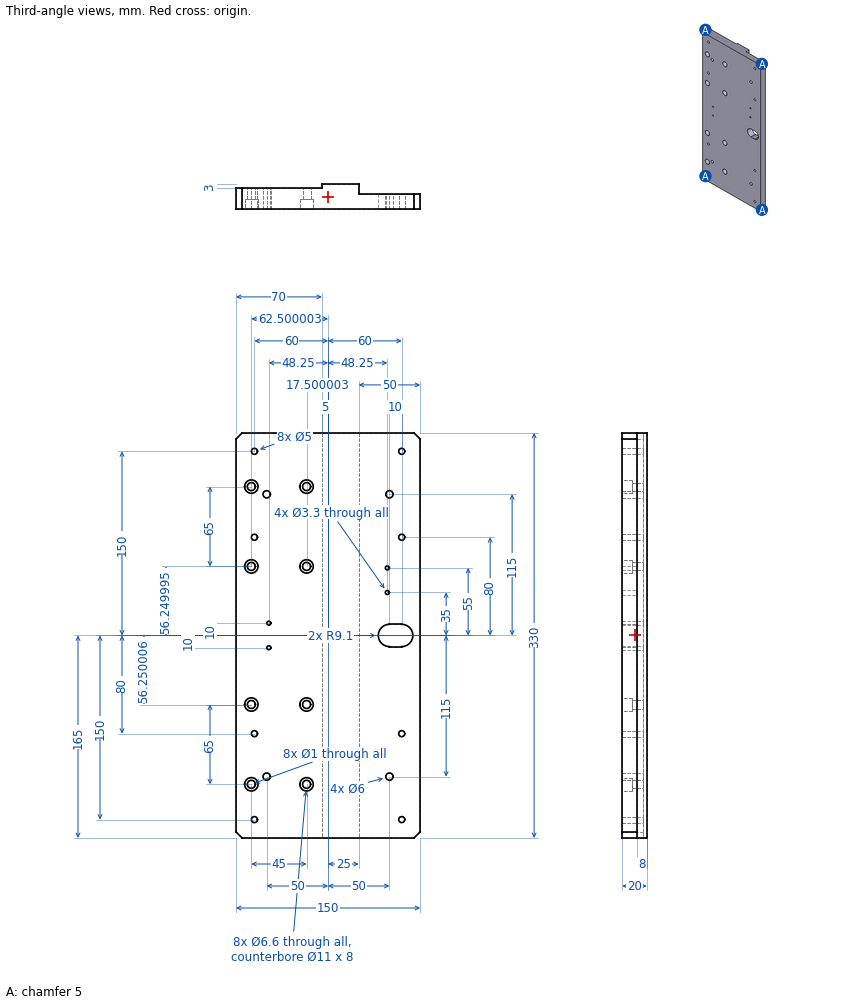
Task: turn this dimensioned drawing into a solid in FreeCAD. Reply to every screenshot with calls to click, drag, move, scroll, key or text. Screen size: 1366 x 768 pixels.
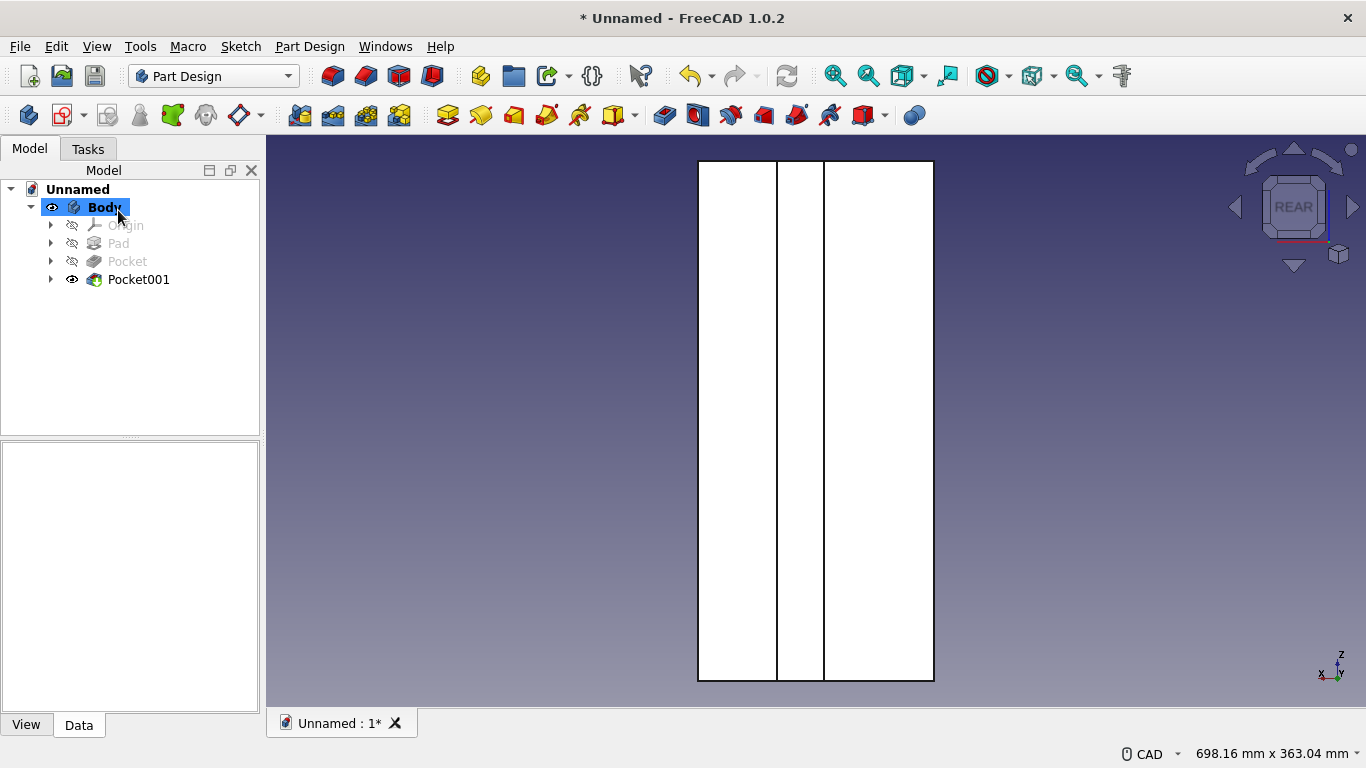
click(879, 569)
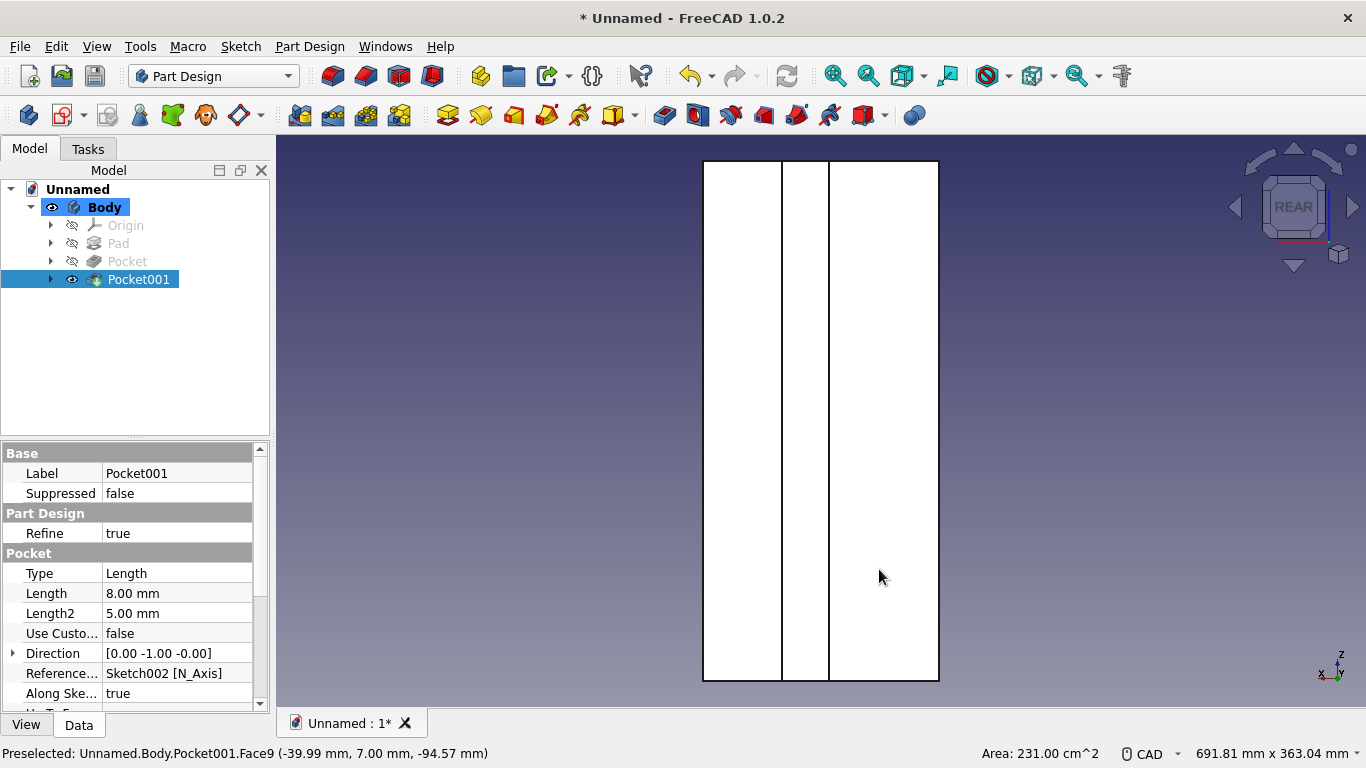
click(62, 116)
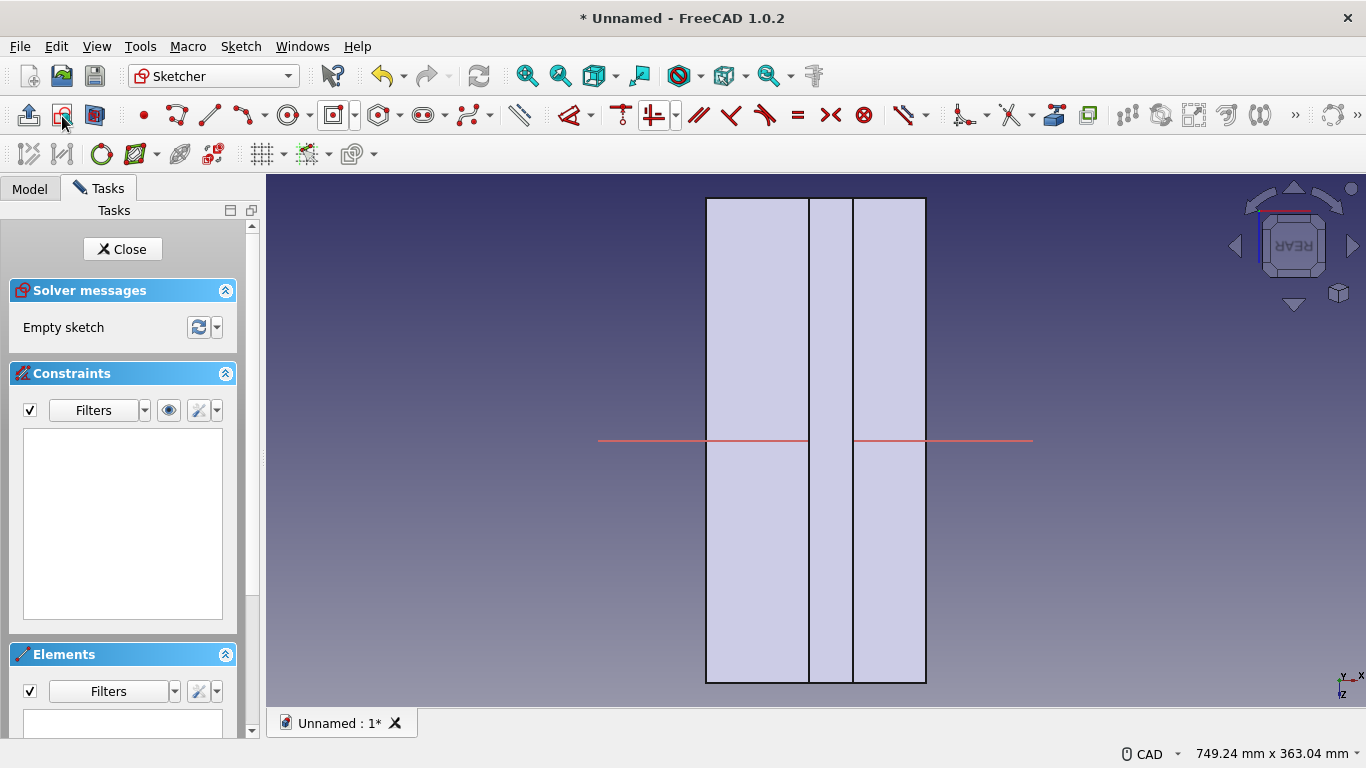
click(95, 116)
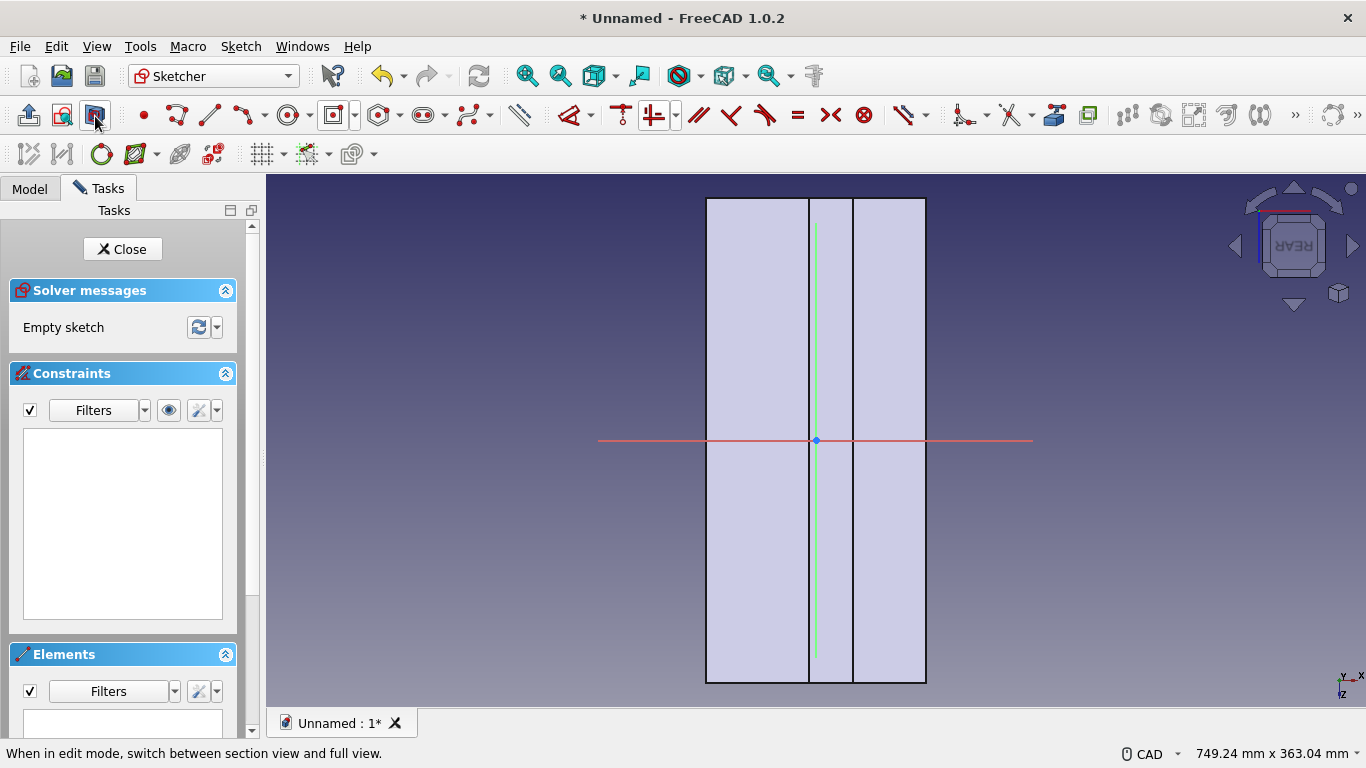
click(288, 116)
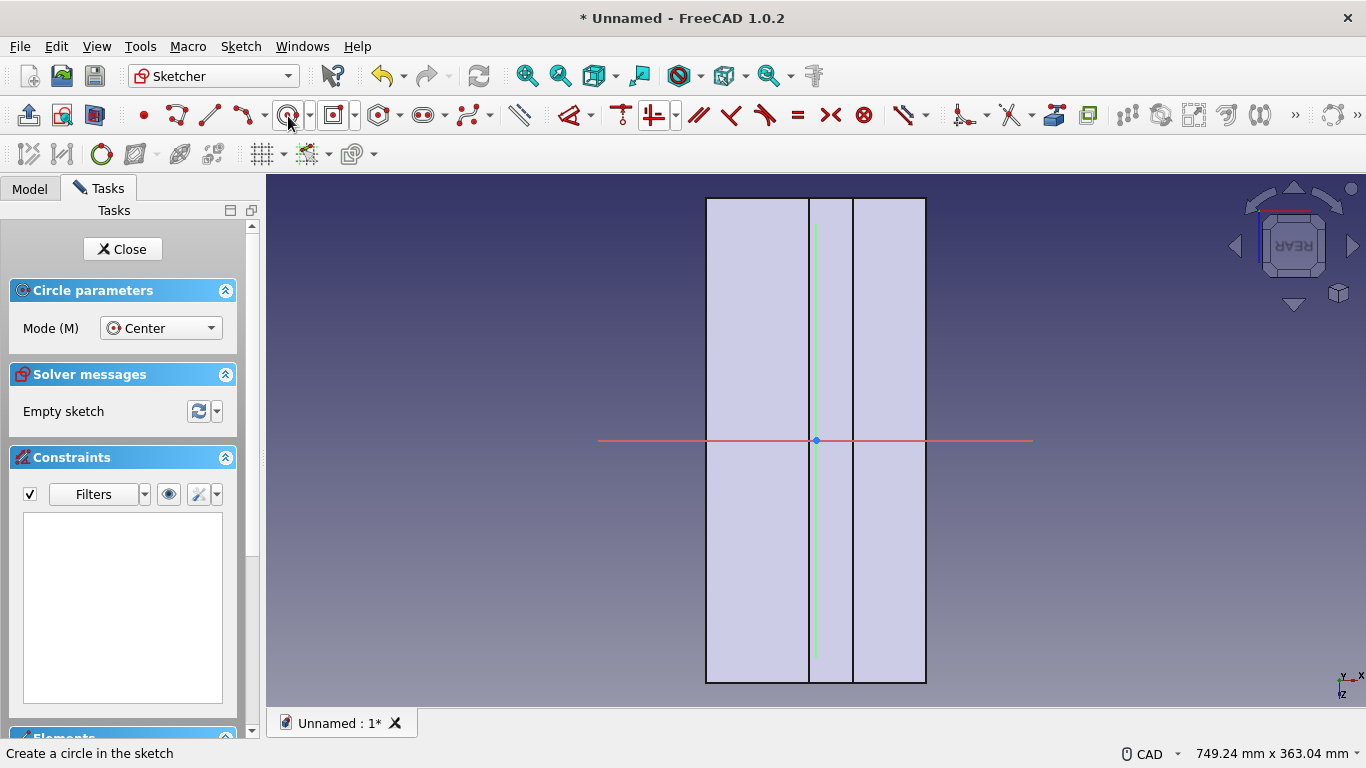
scroll(724, 262, up, 18)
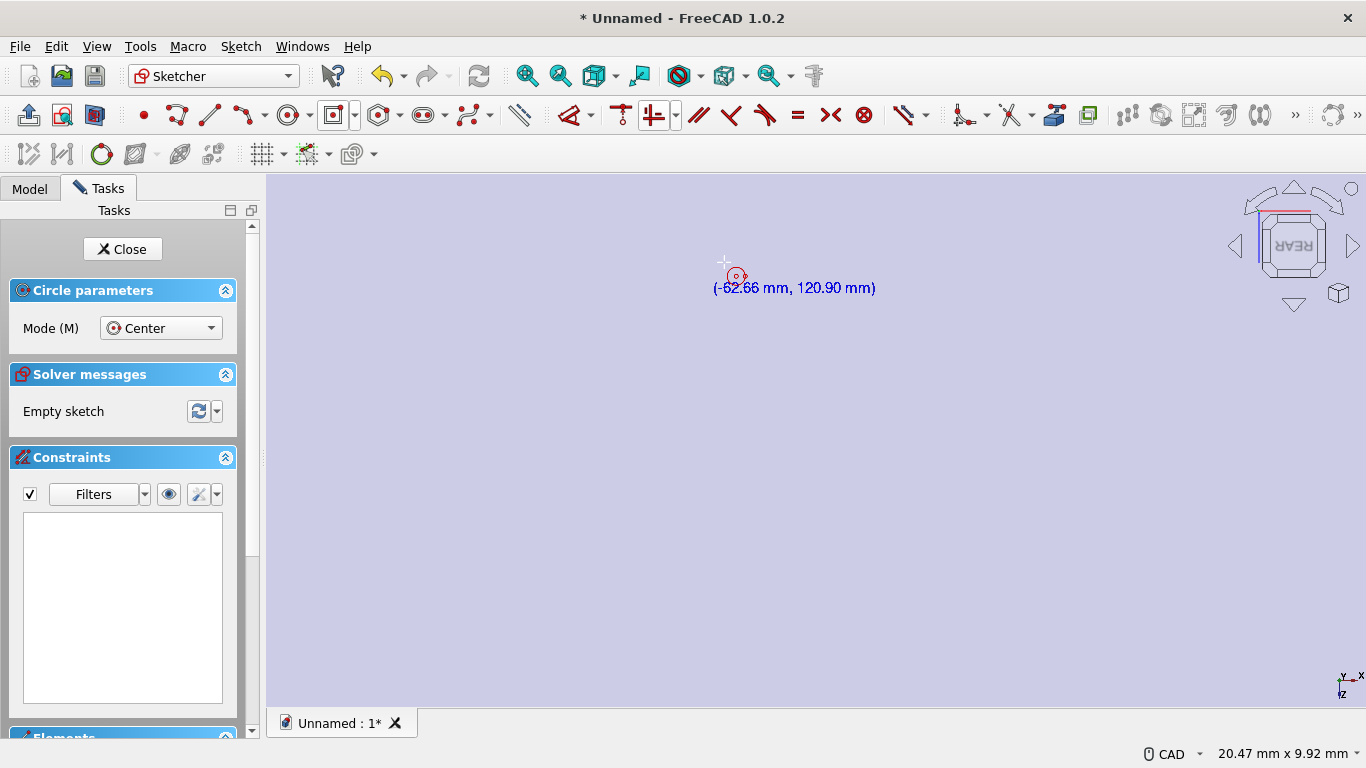
scroll(702, 262, down, 18)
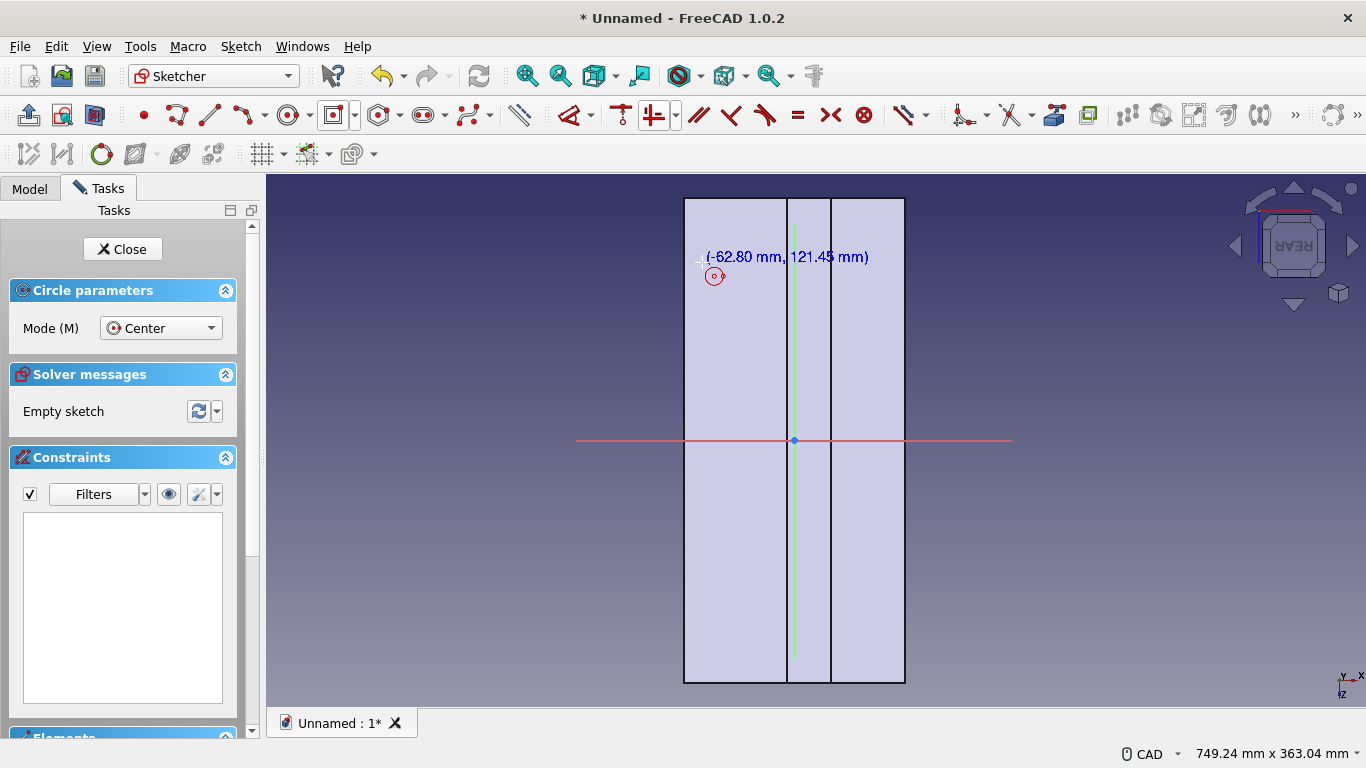
click(703, 262)
move(703, 262)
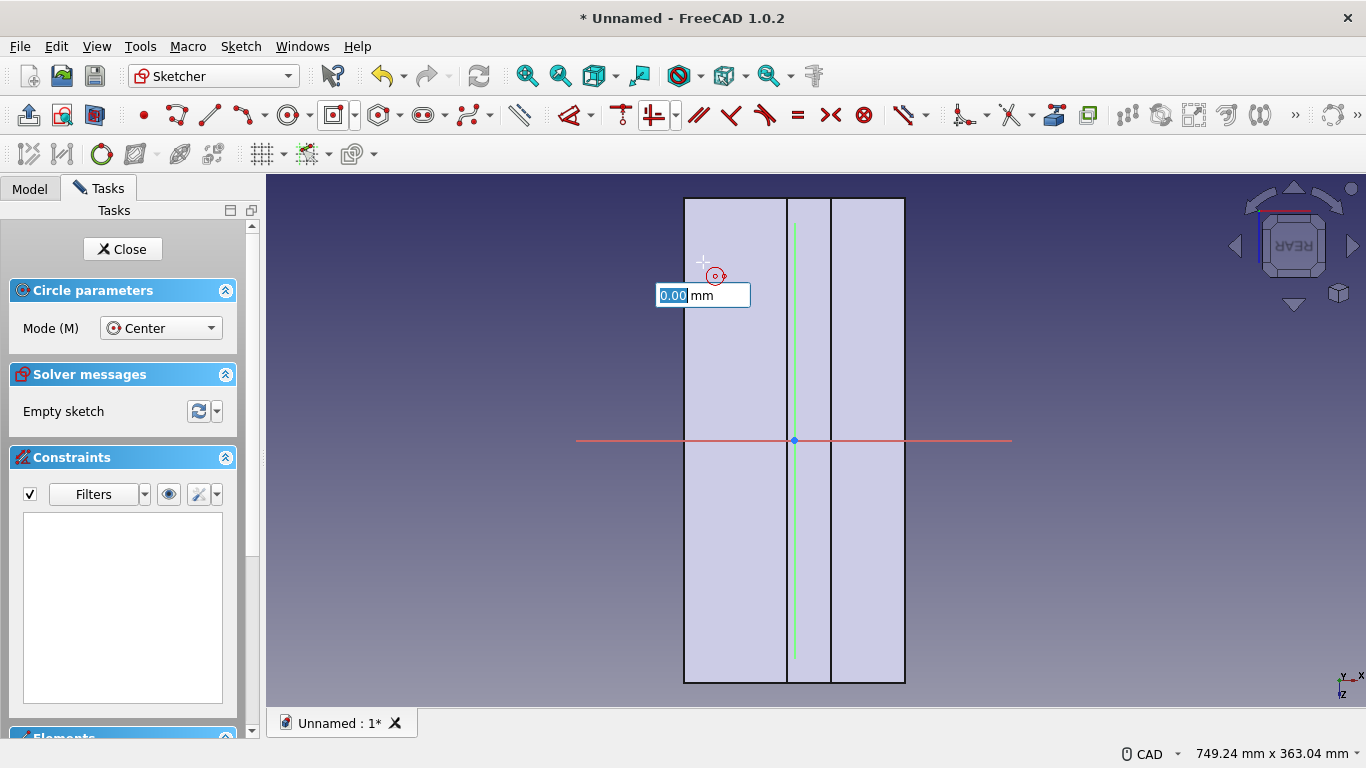
text(1)
key(Return)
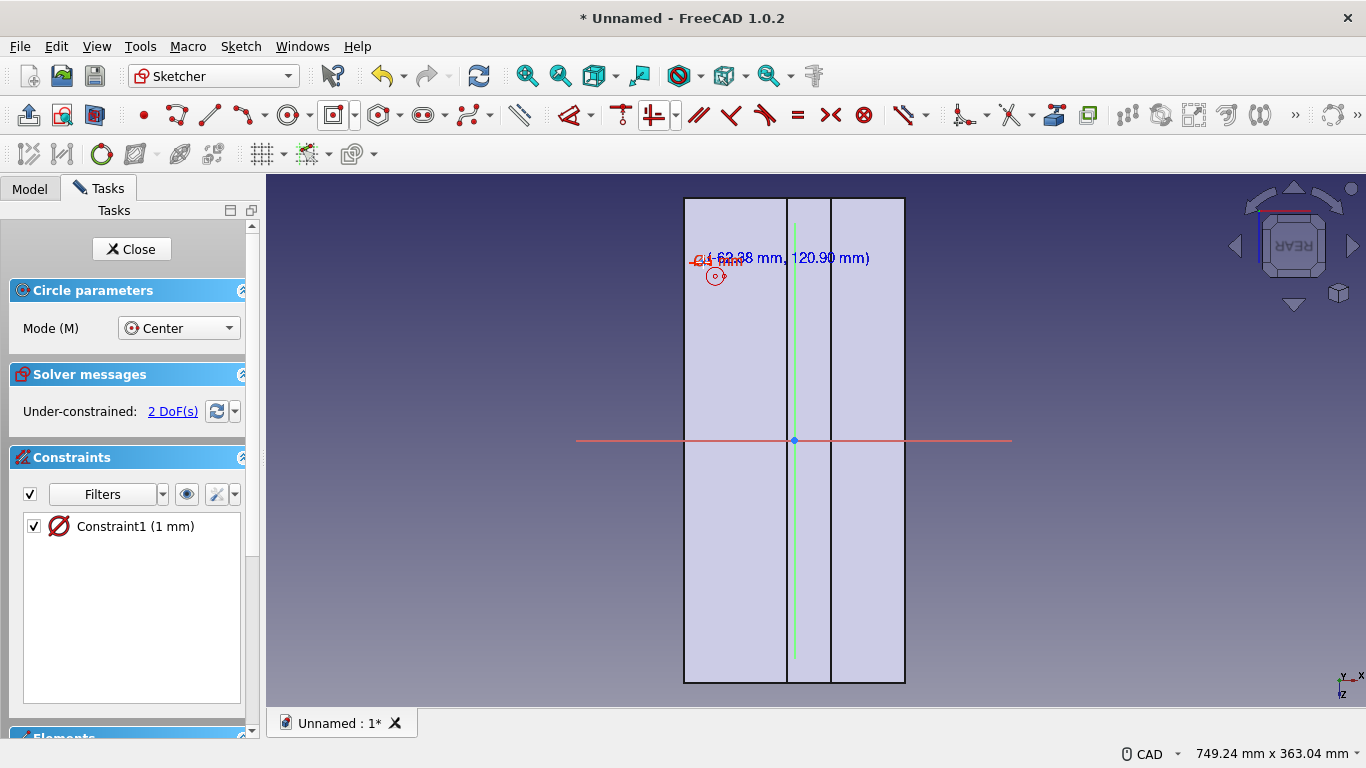
scroll(769, 262, up, 18)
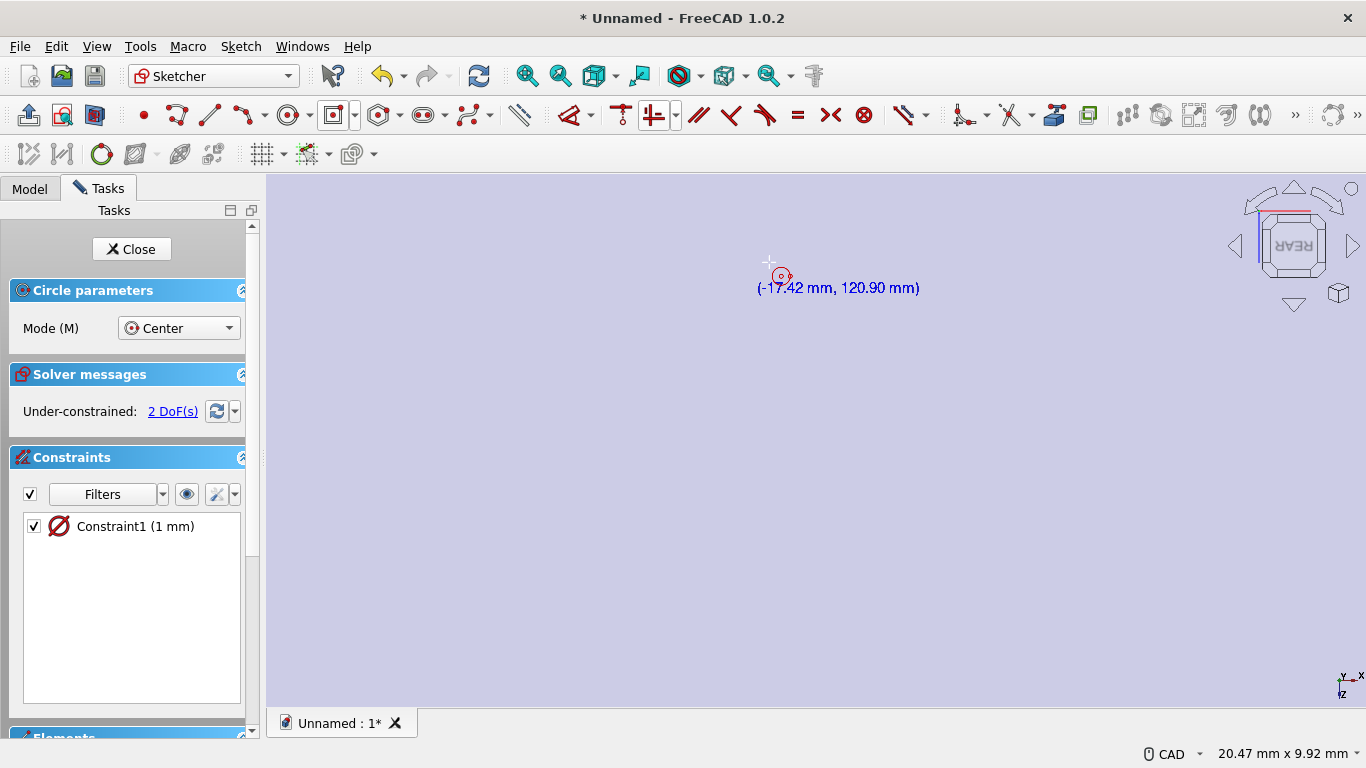
scroll(769, 262, down, 18)